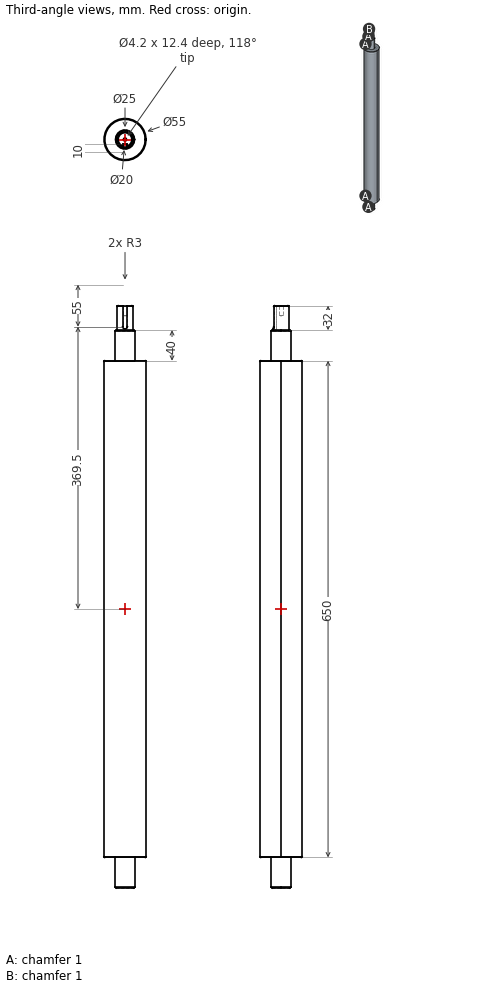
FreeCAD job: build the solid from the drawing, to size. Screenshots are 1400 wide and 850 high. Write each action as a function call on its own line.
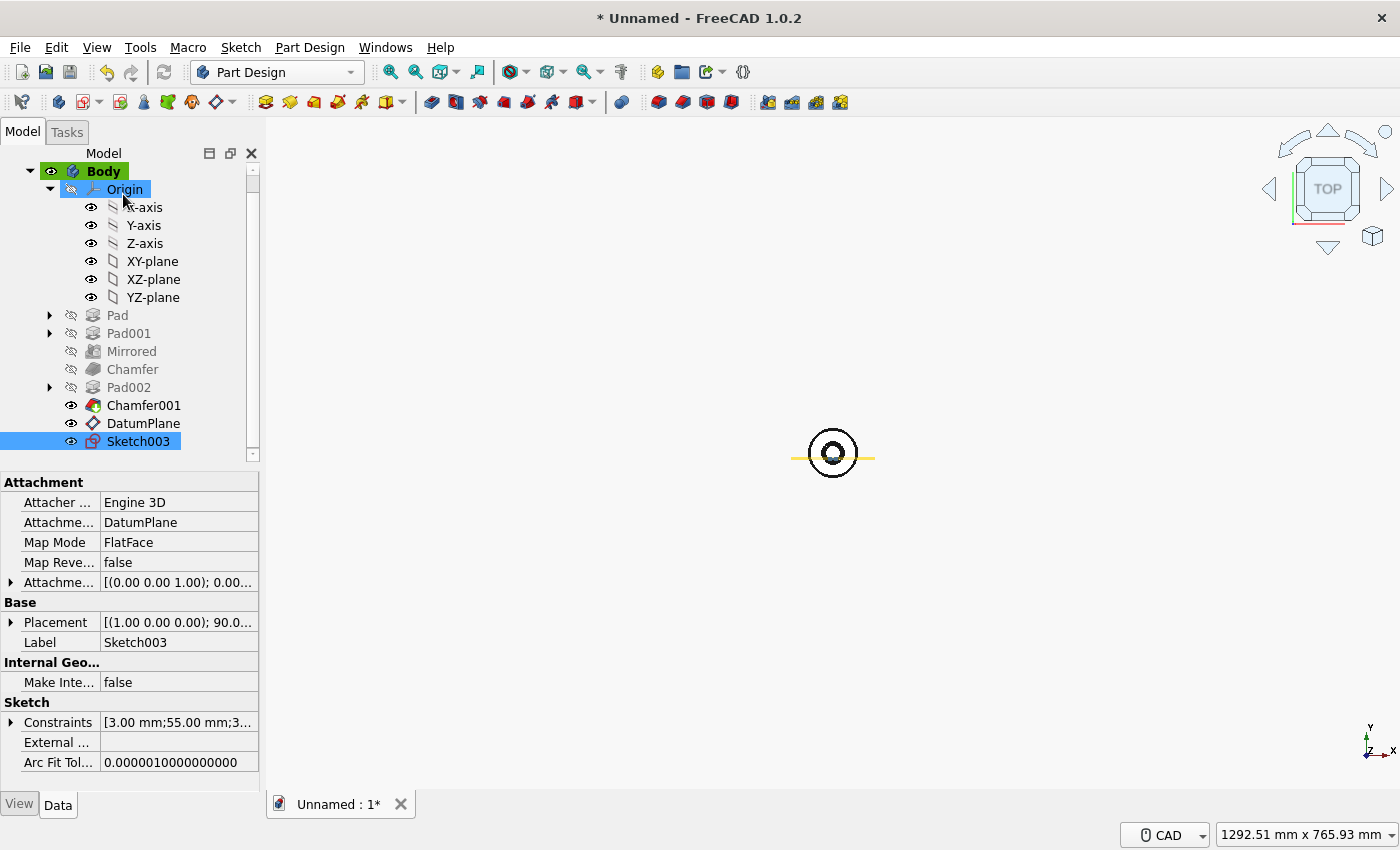
click(432, 102)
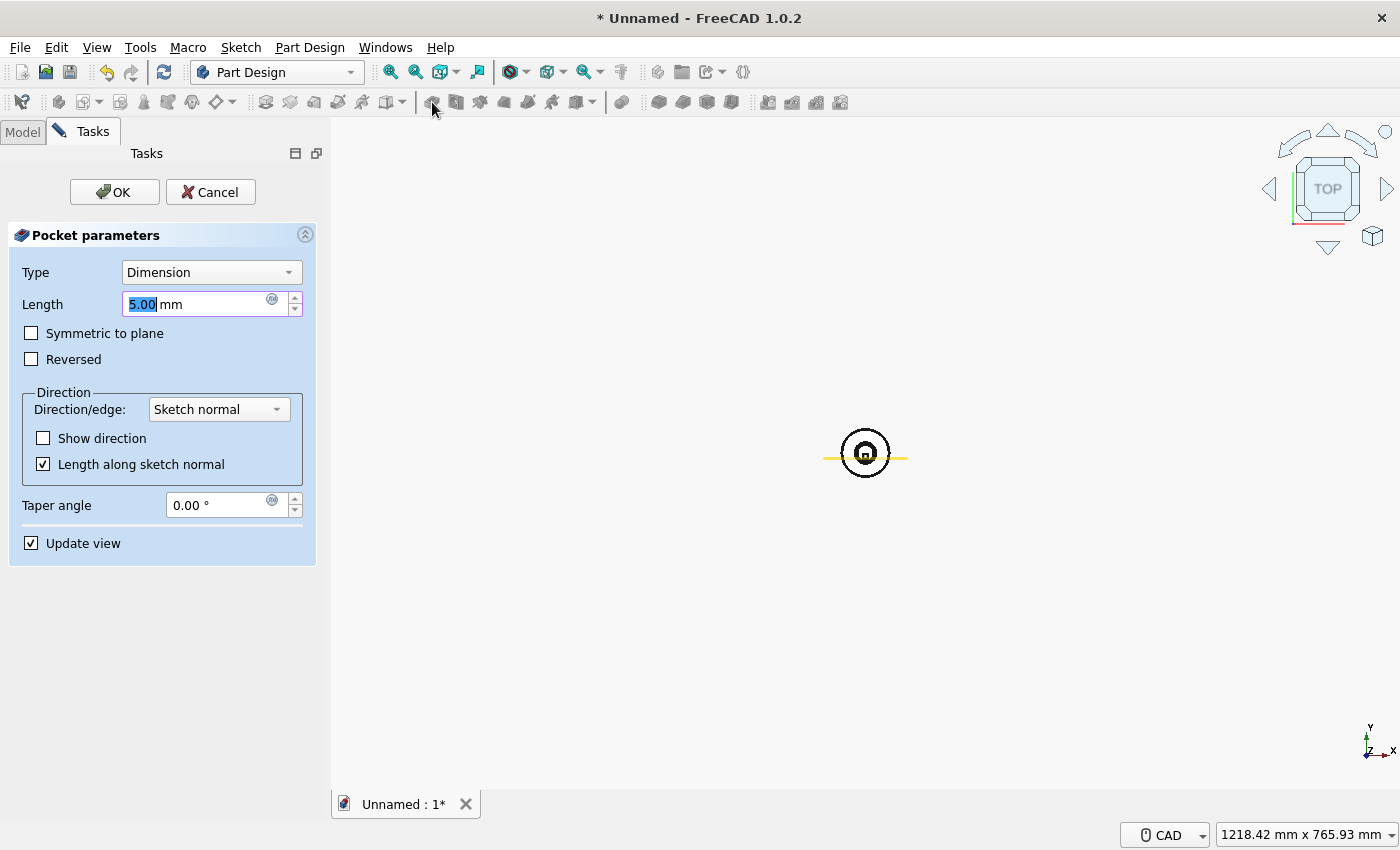
text(10)
key(Tab)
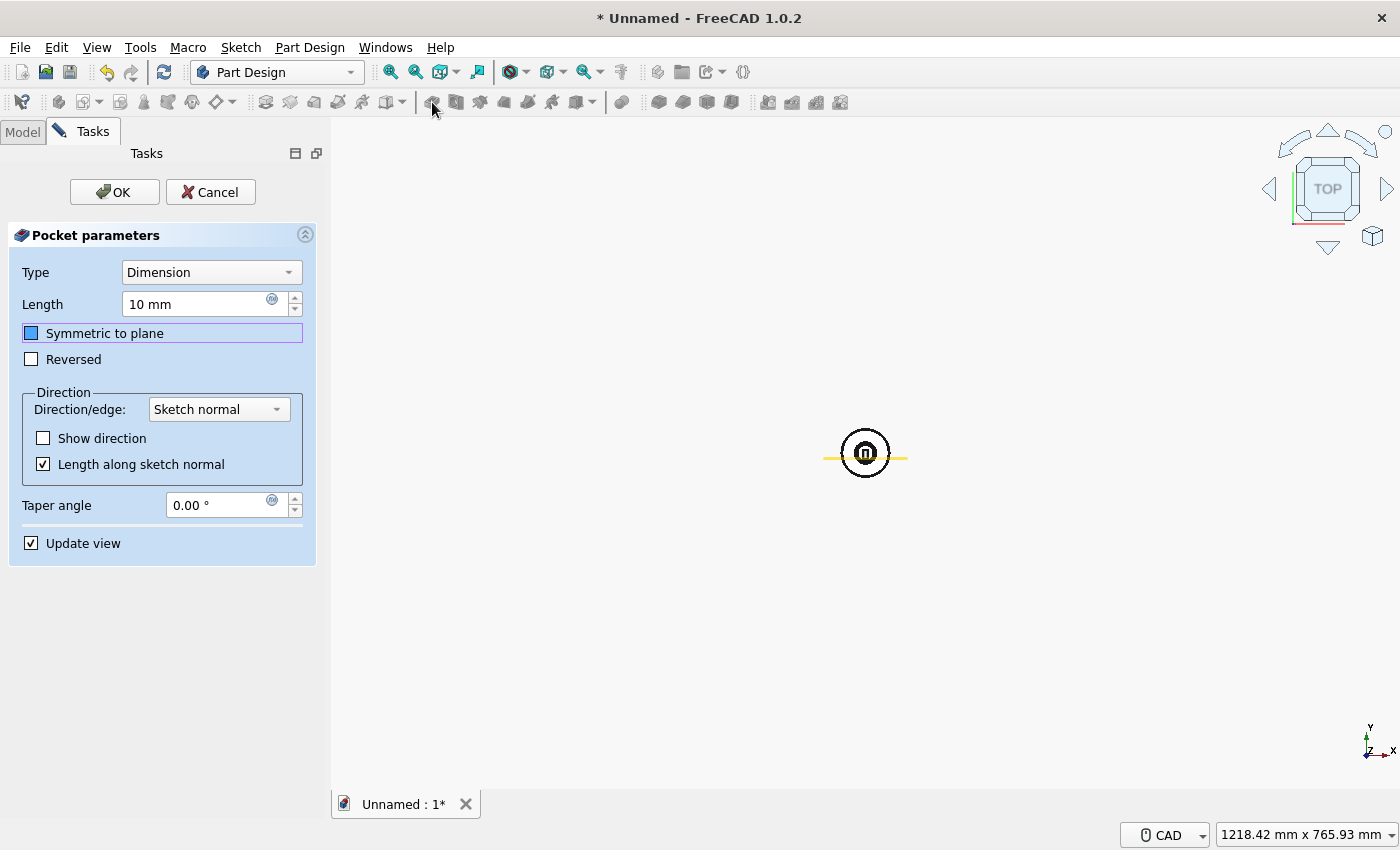
click(30, 359)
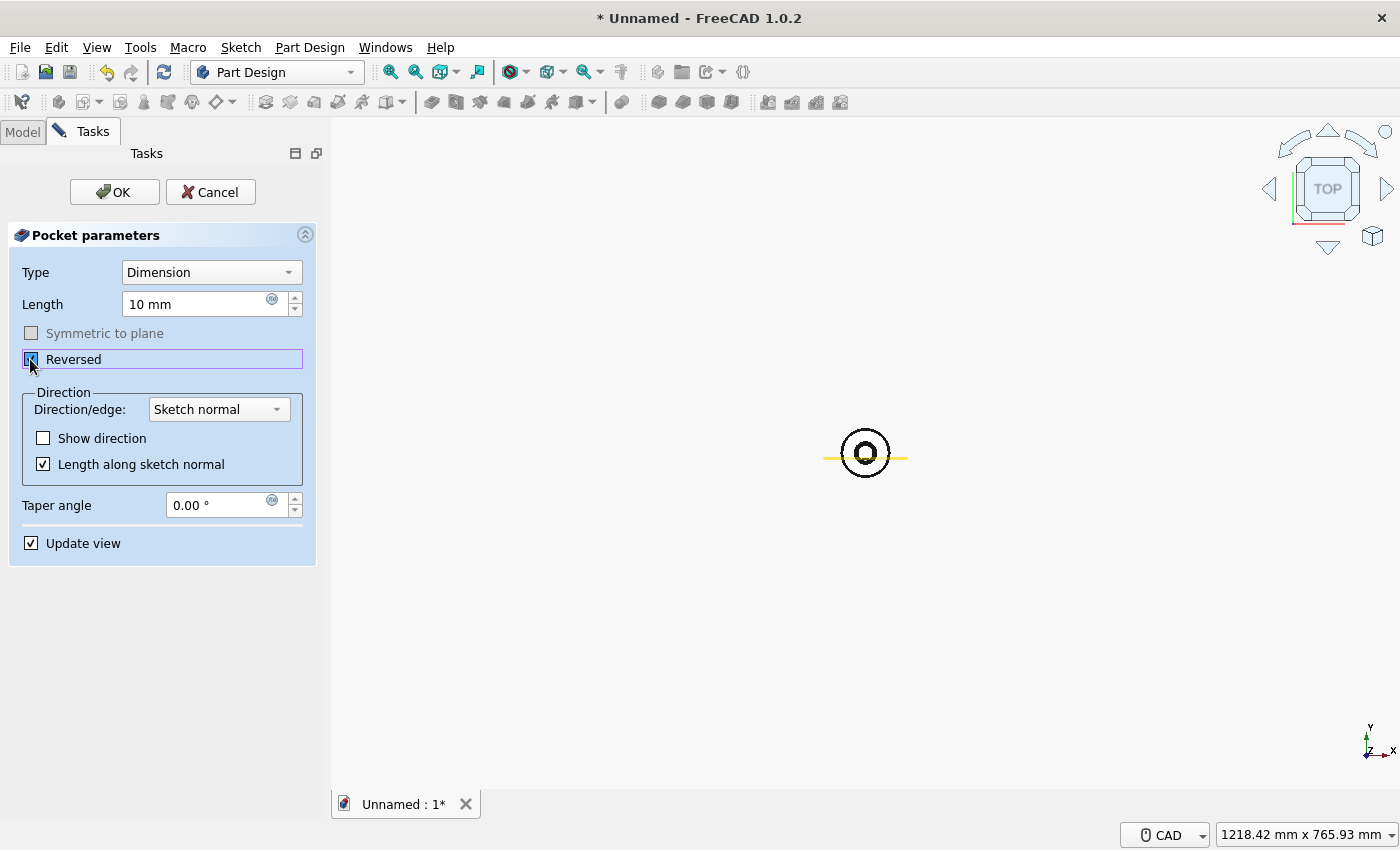
click(115, 192)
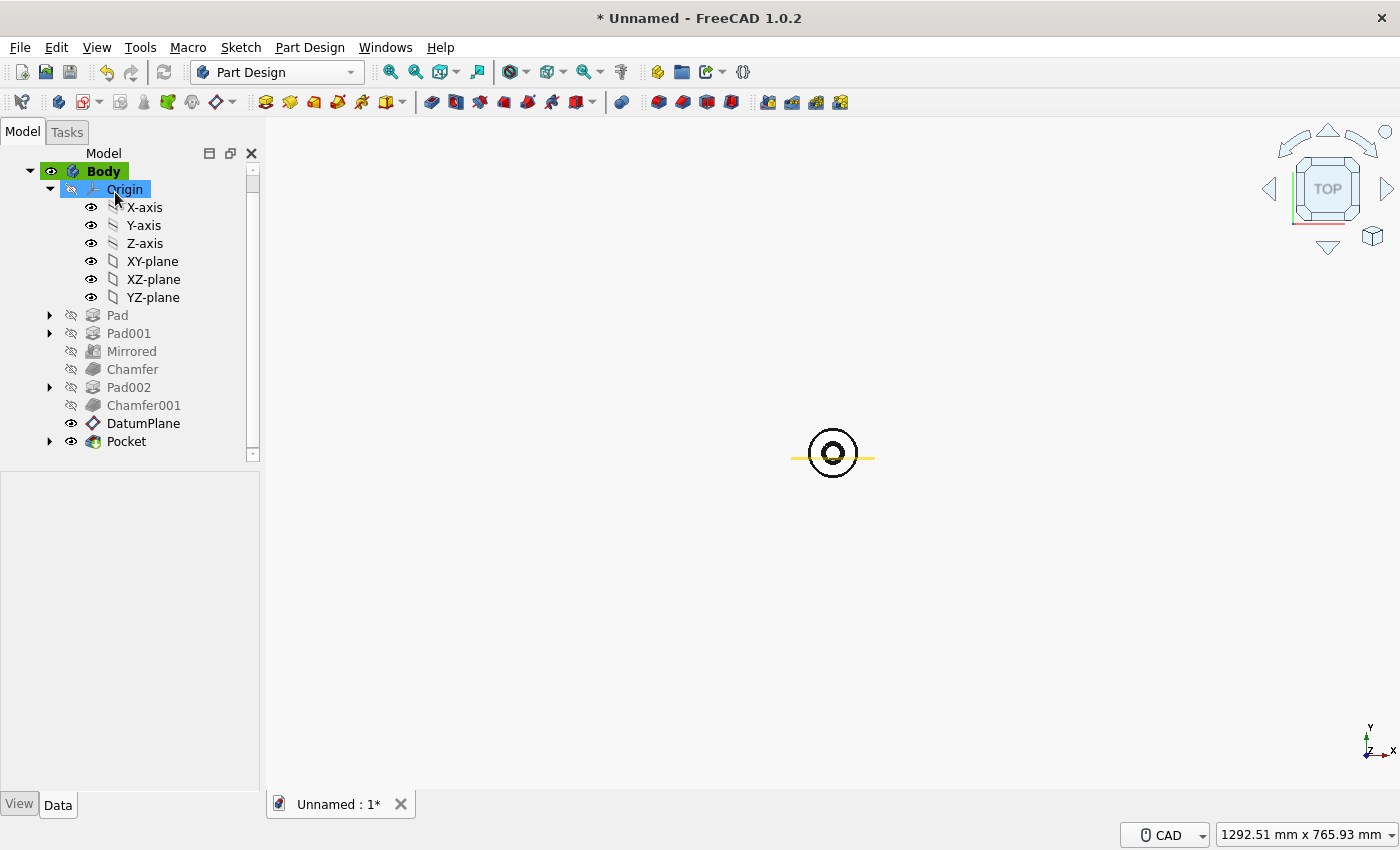
click(116, 423)
key(space)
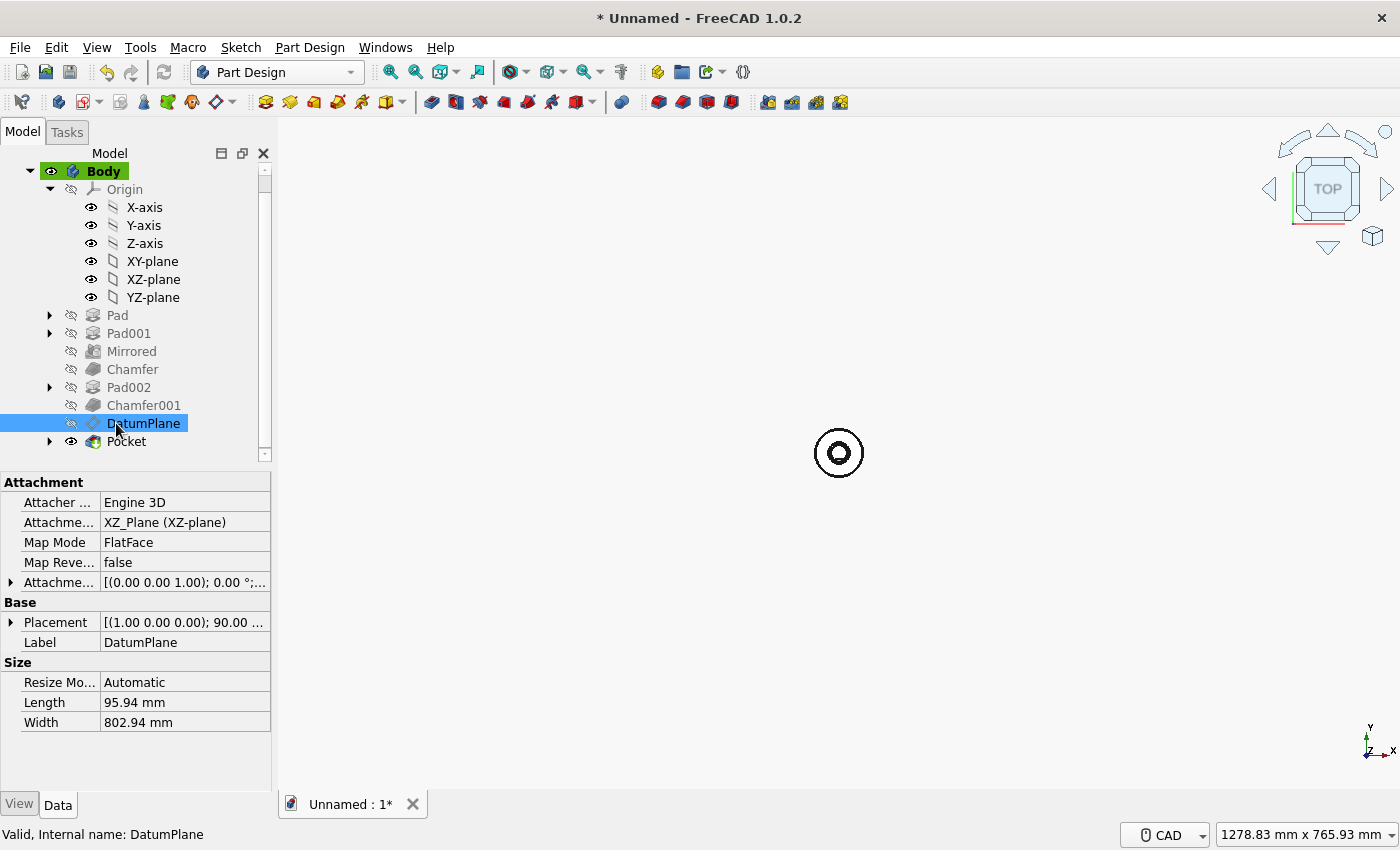
click(392, 72)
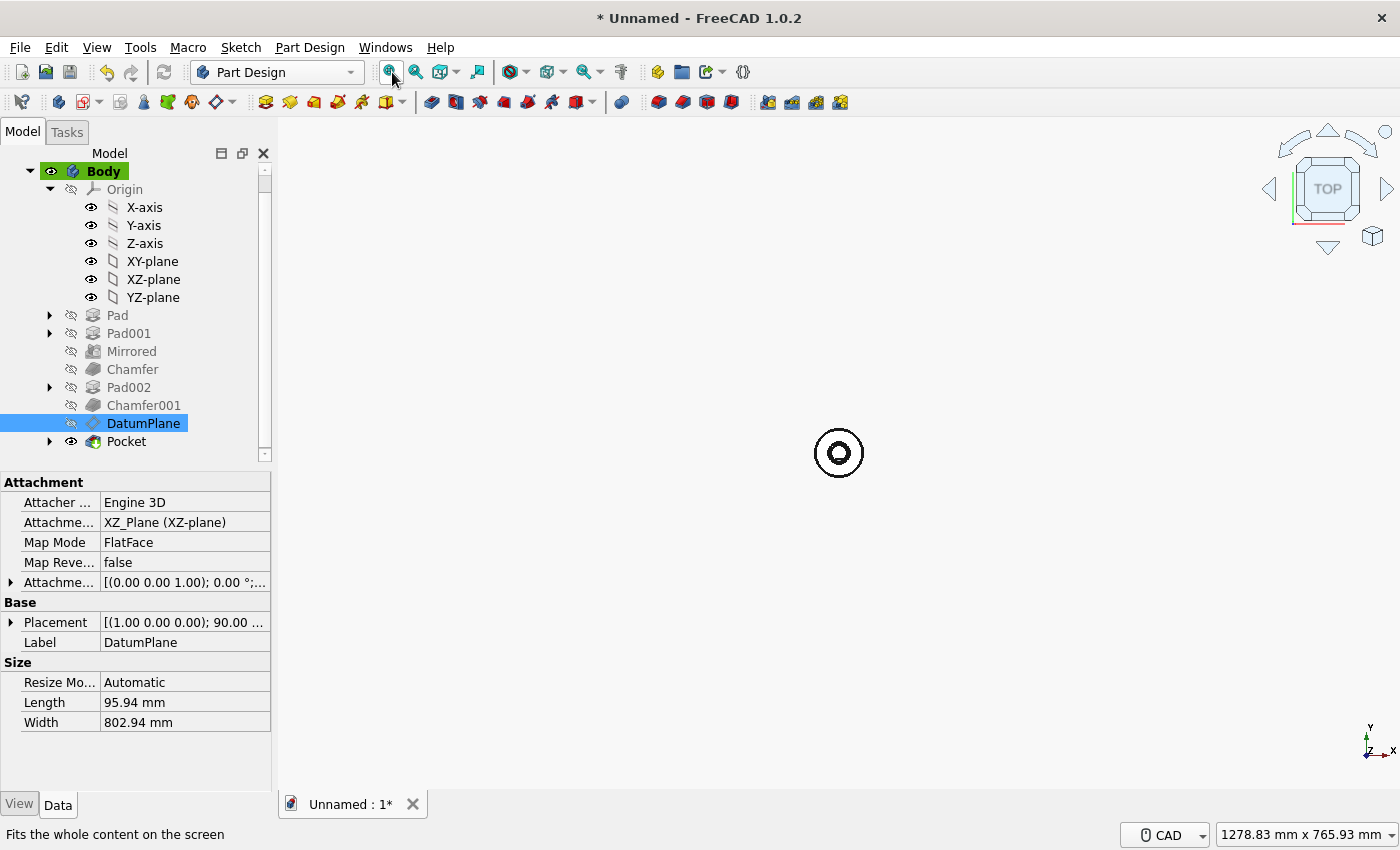
scroll(839, 452, up, 4)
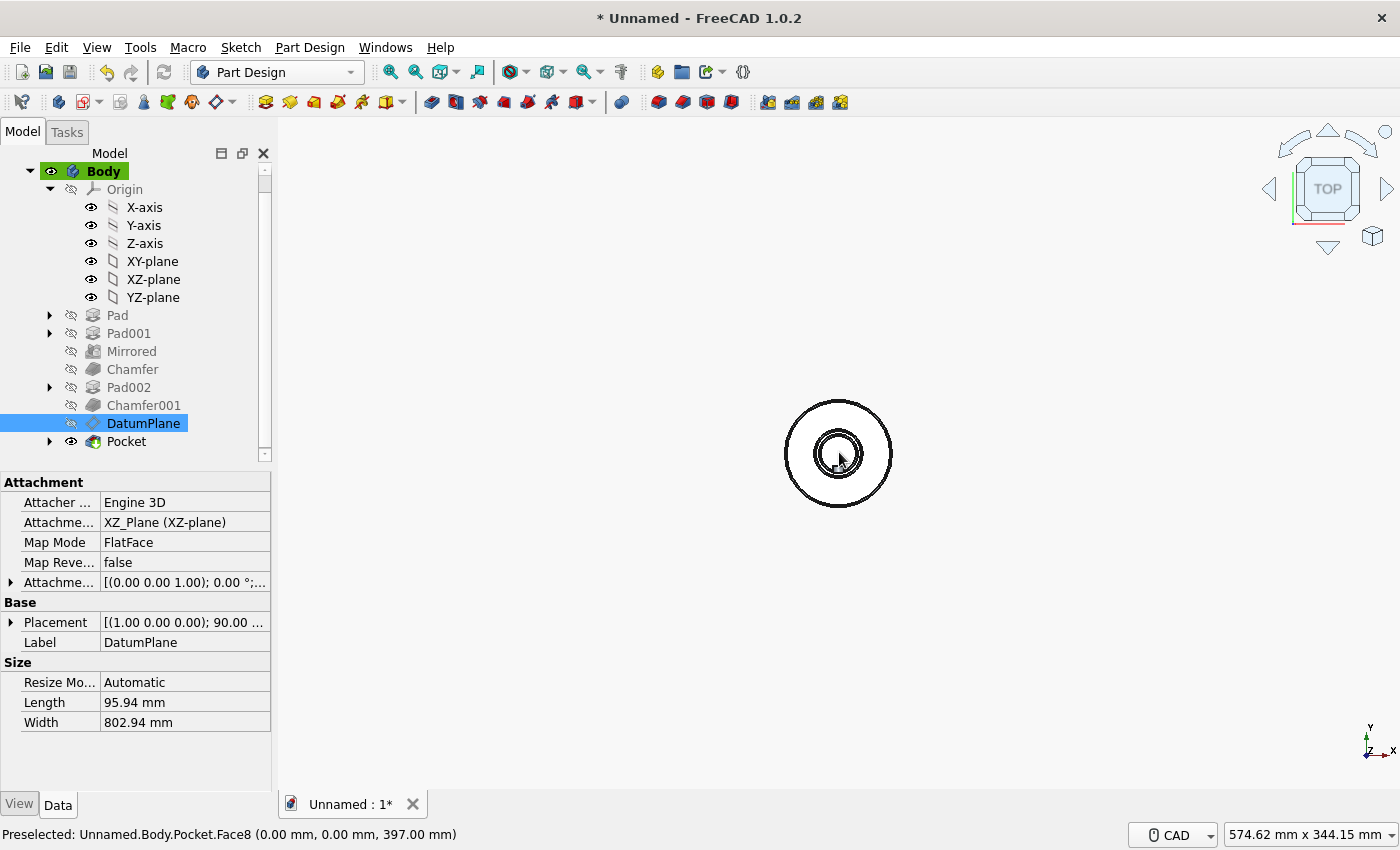
click(838, 452)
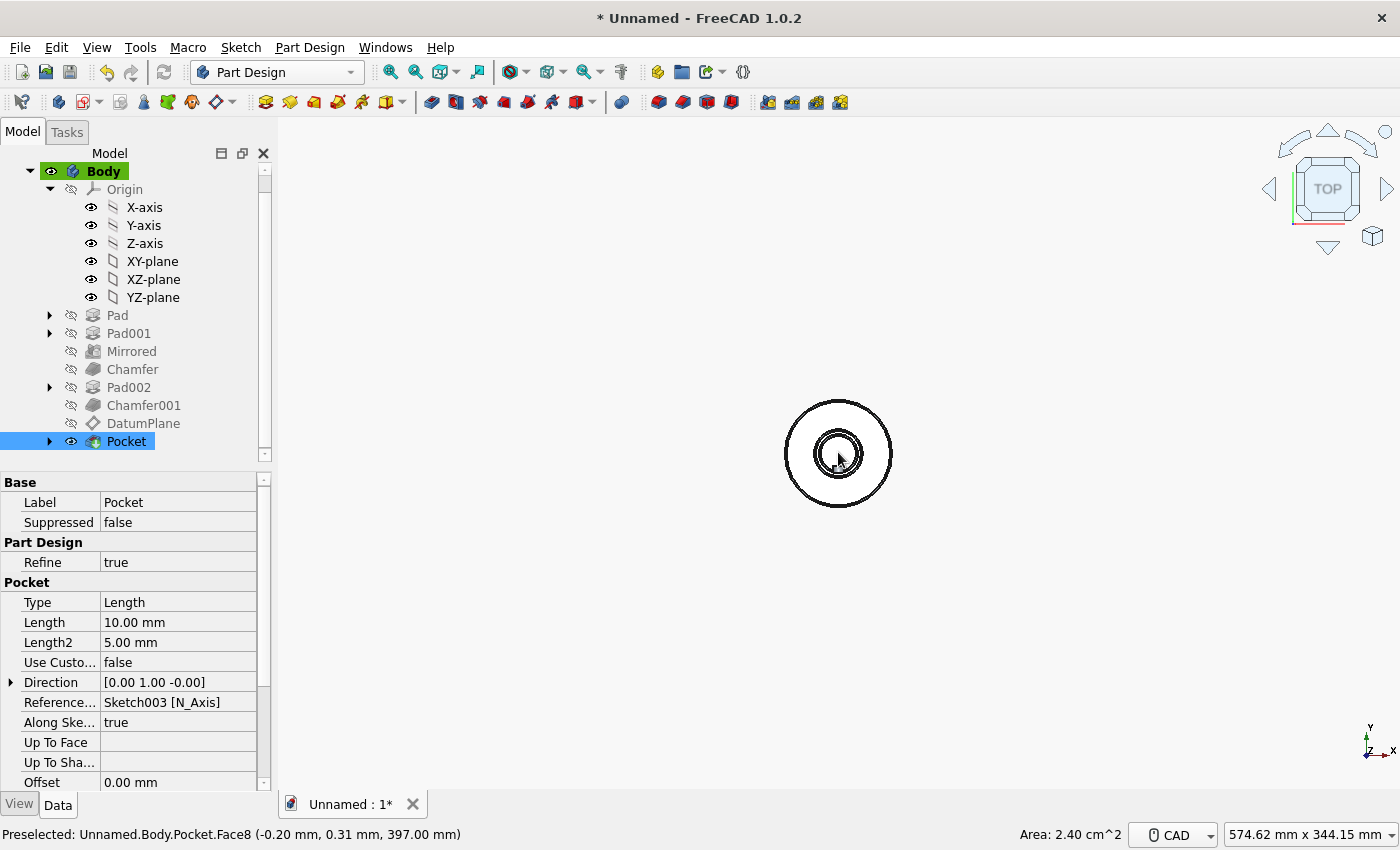
click(84, 102)